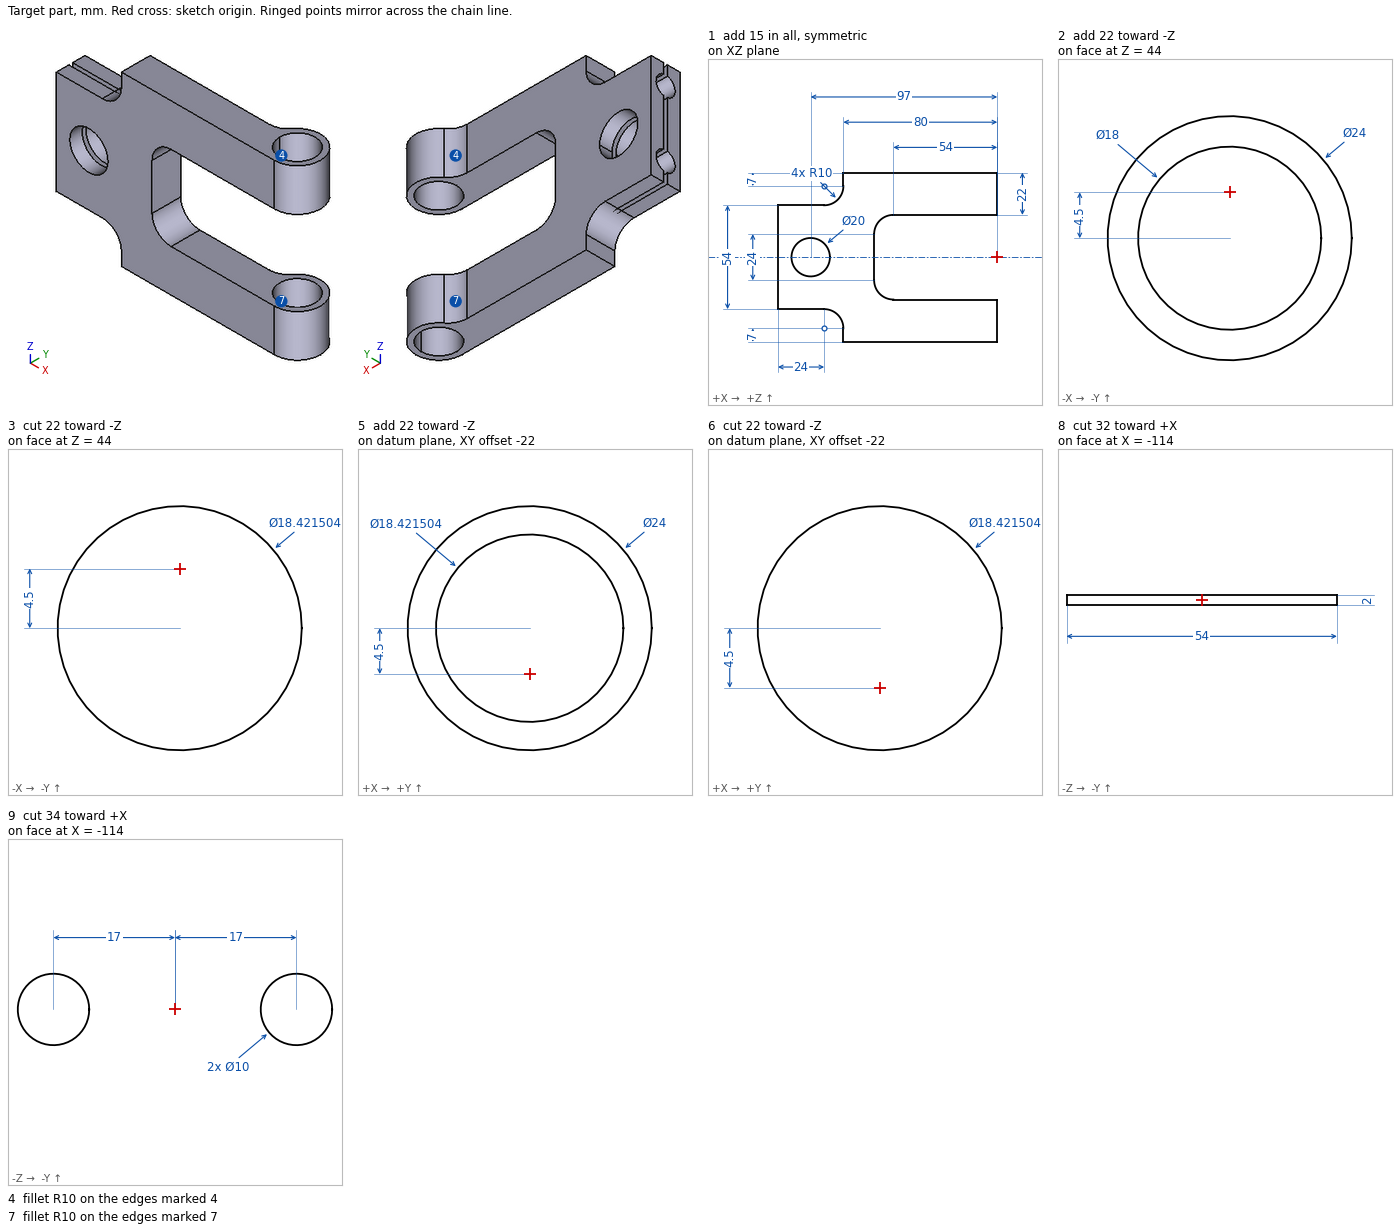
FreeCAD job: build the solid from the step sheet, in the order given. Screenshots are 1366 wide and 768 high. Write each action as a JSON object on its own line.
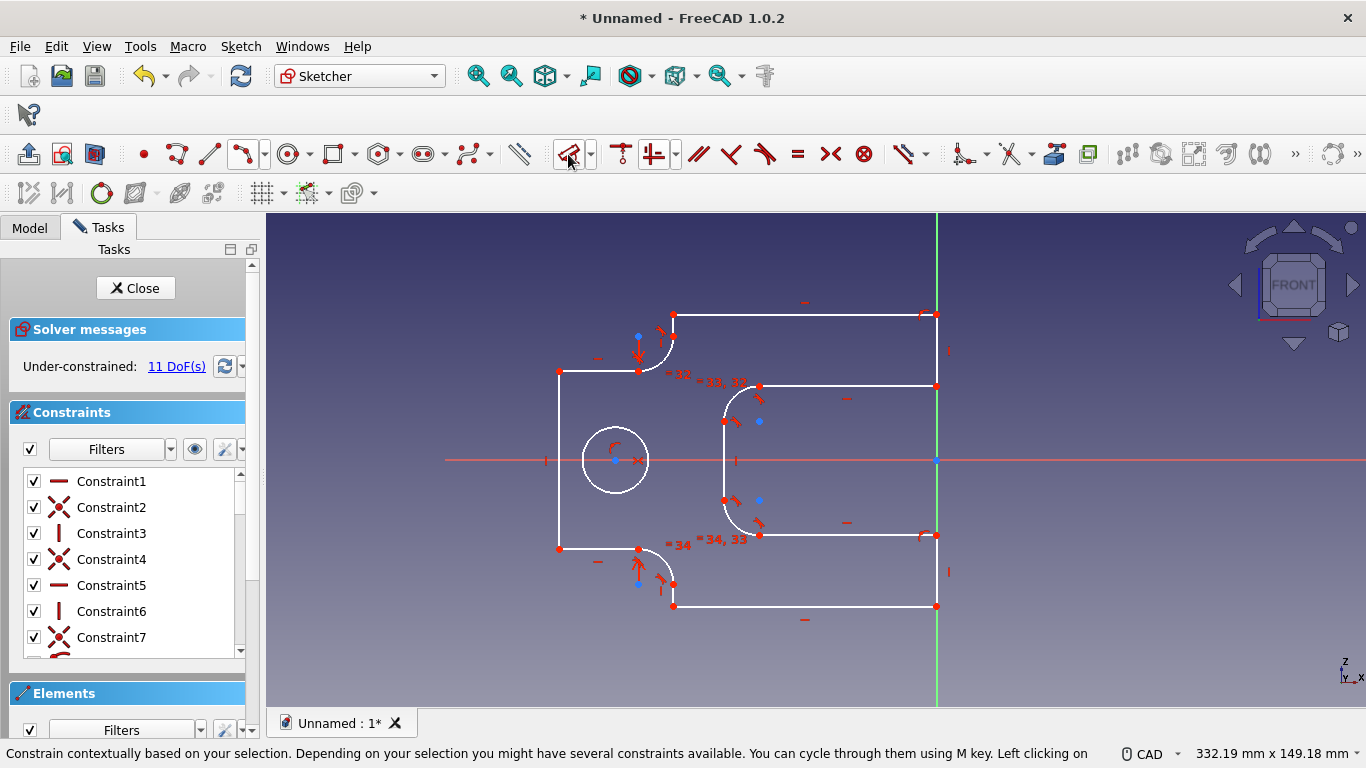
{"action": "left_click", "coordinate": [654, 367]}
{"action": "left_click", "coordinate": [668, 396]}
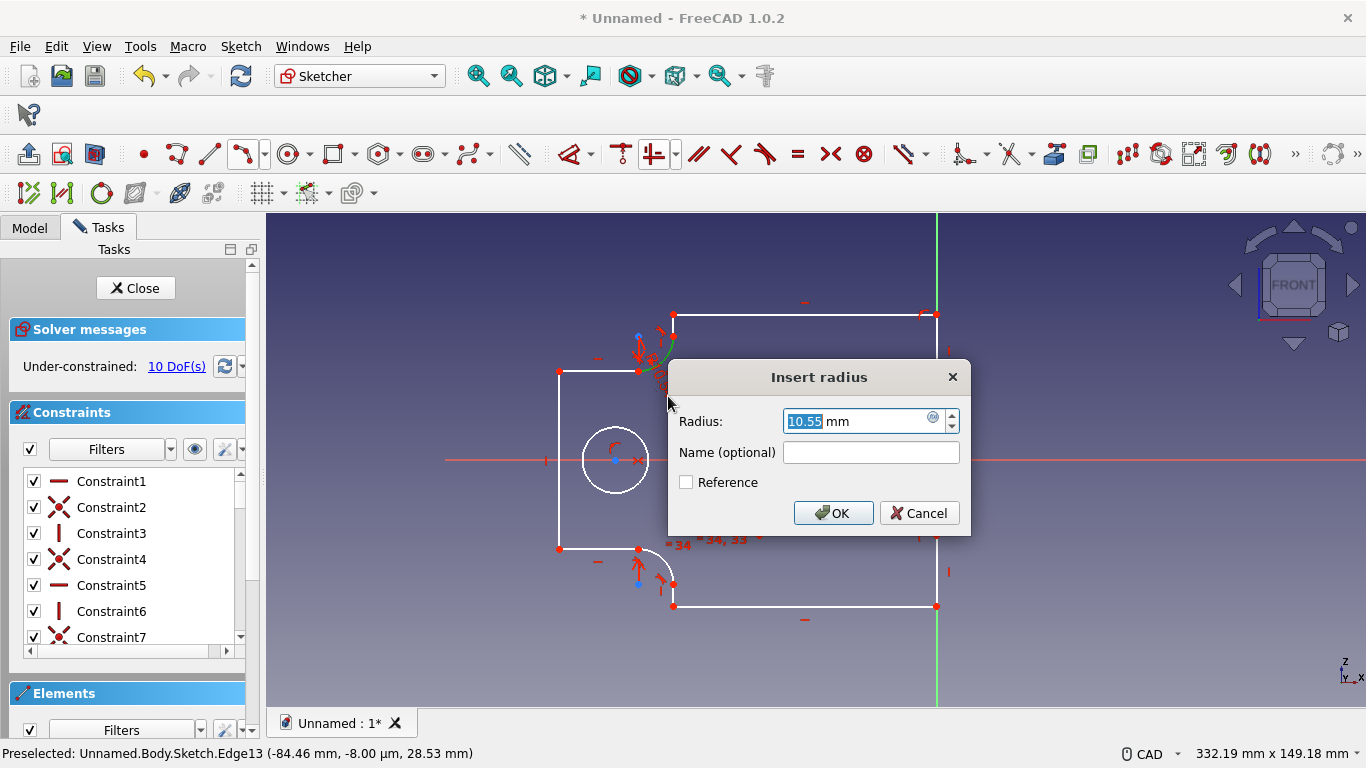
{"action": "type", "text": "10"}
{"action": "key", "text": "Return"}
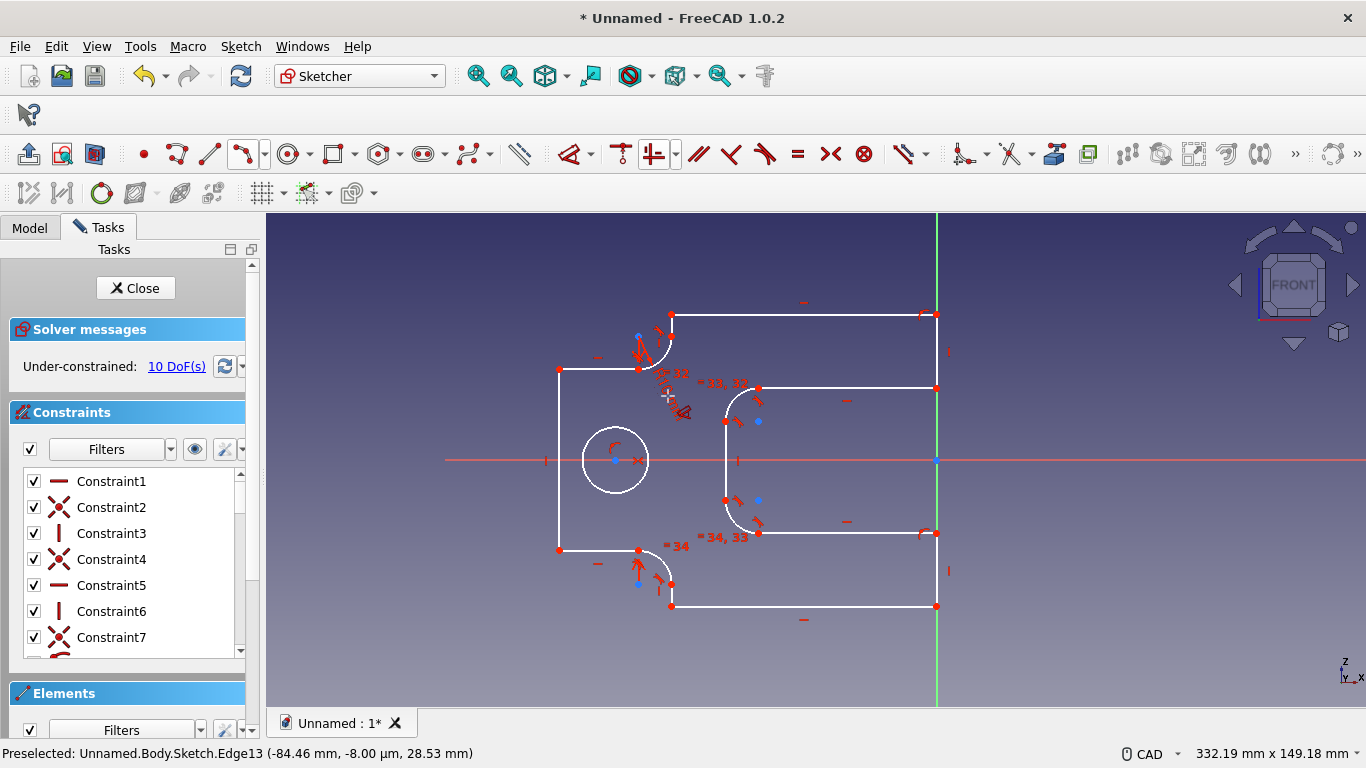
{"action": "left_click", "coordinate": [639, 437]}
{"action": "left_click", "coordinate": [678, 442]}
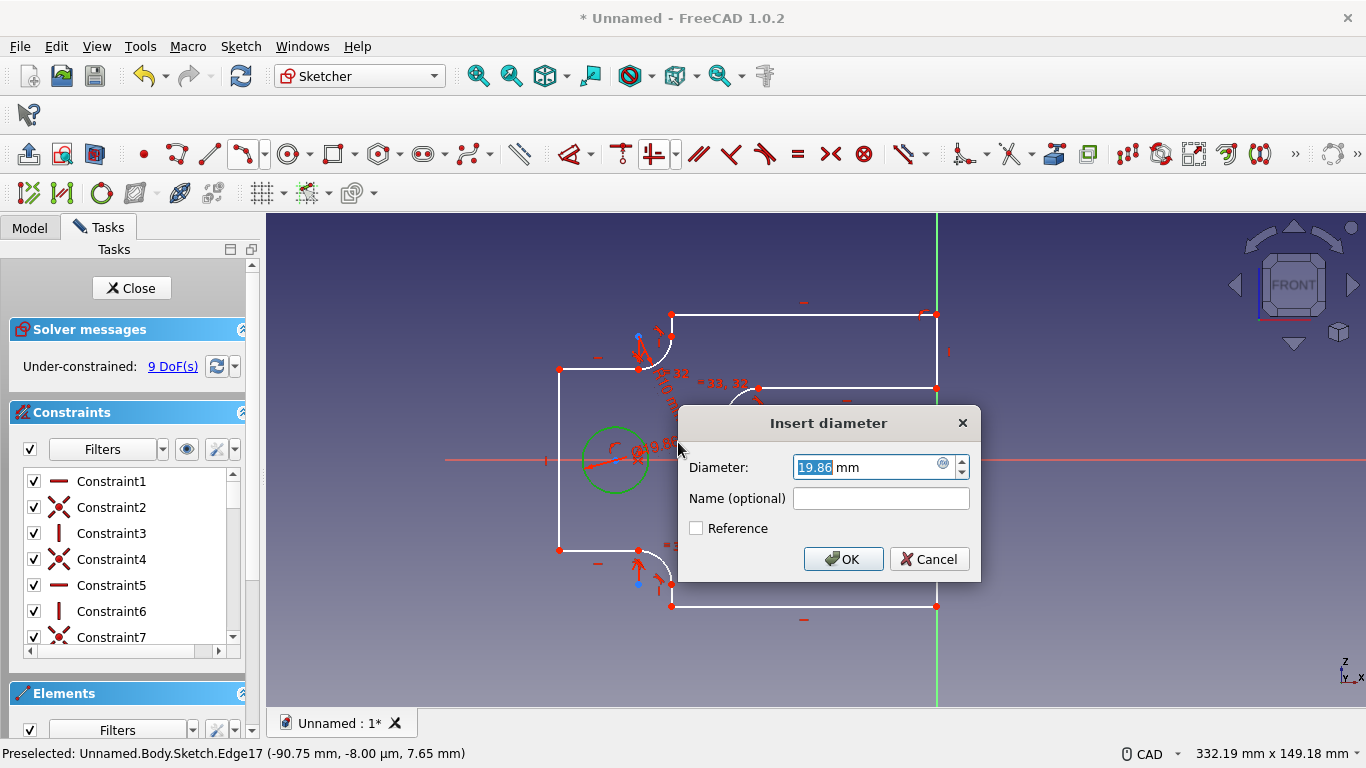
{"action": "type", "text": "20"}
{"action": "key", "text": "Return"}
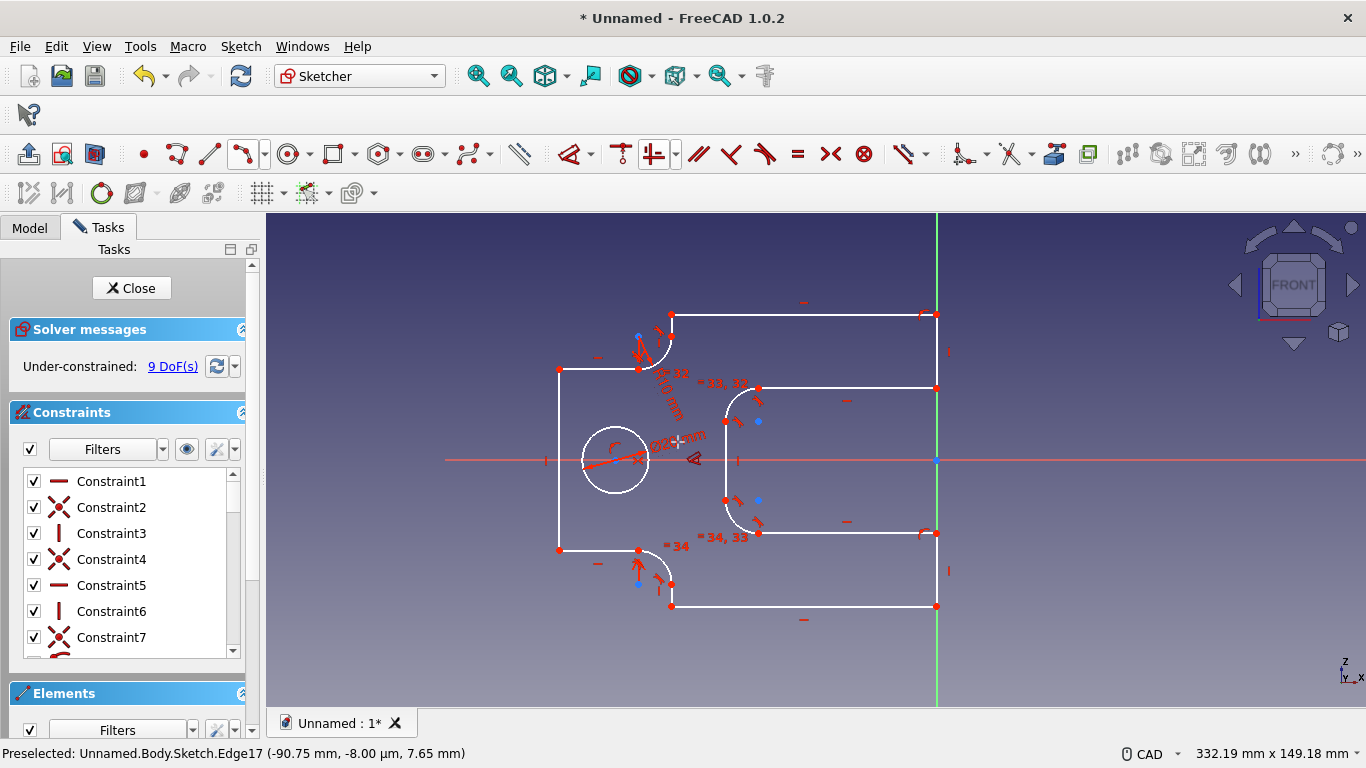
{"action": "scroll", "coordinate": [672, 326], "scroll_direction": "up", "scroll_amount": 3}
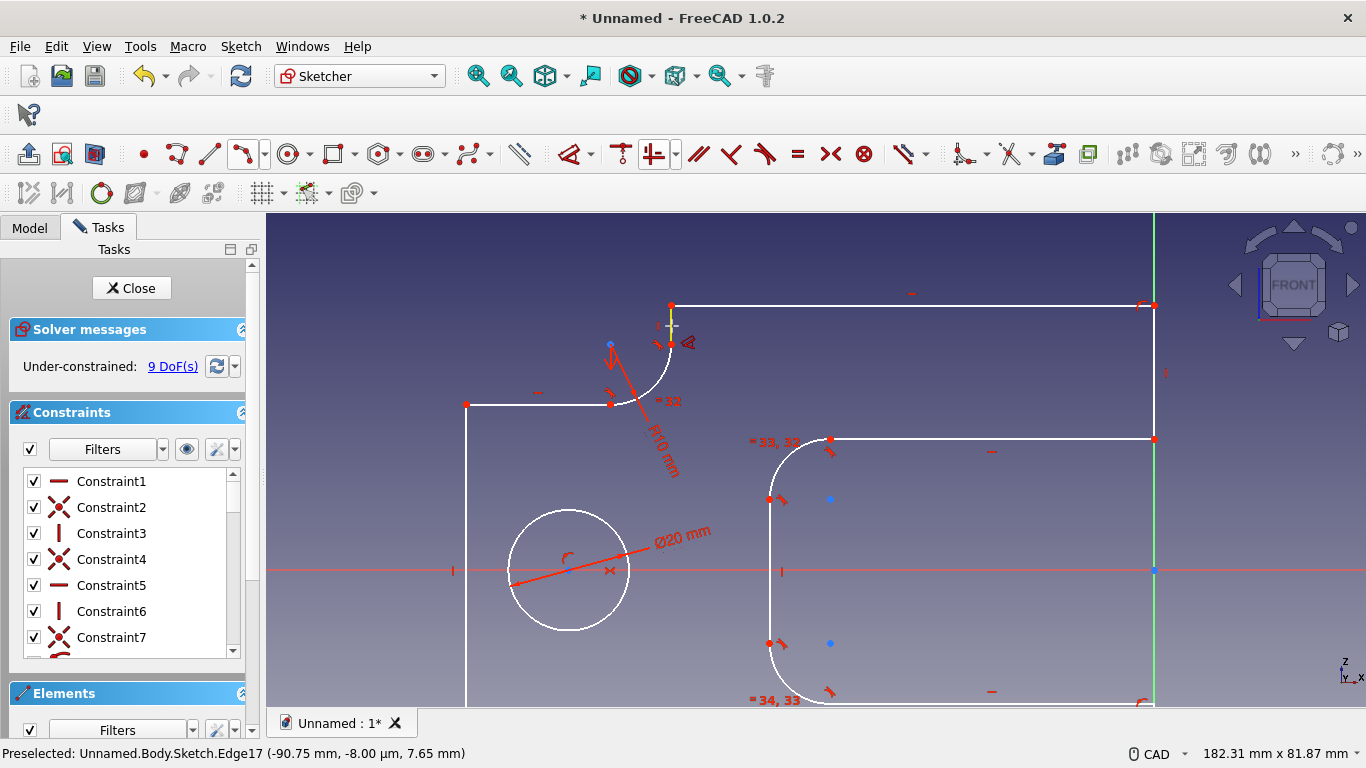
{"action": "left_click", "coordinate": [671, 325]}
{"action": "left_click", "coordinate": [637, 325]}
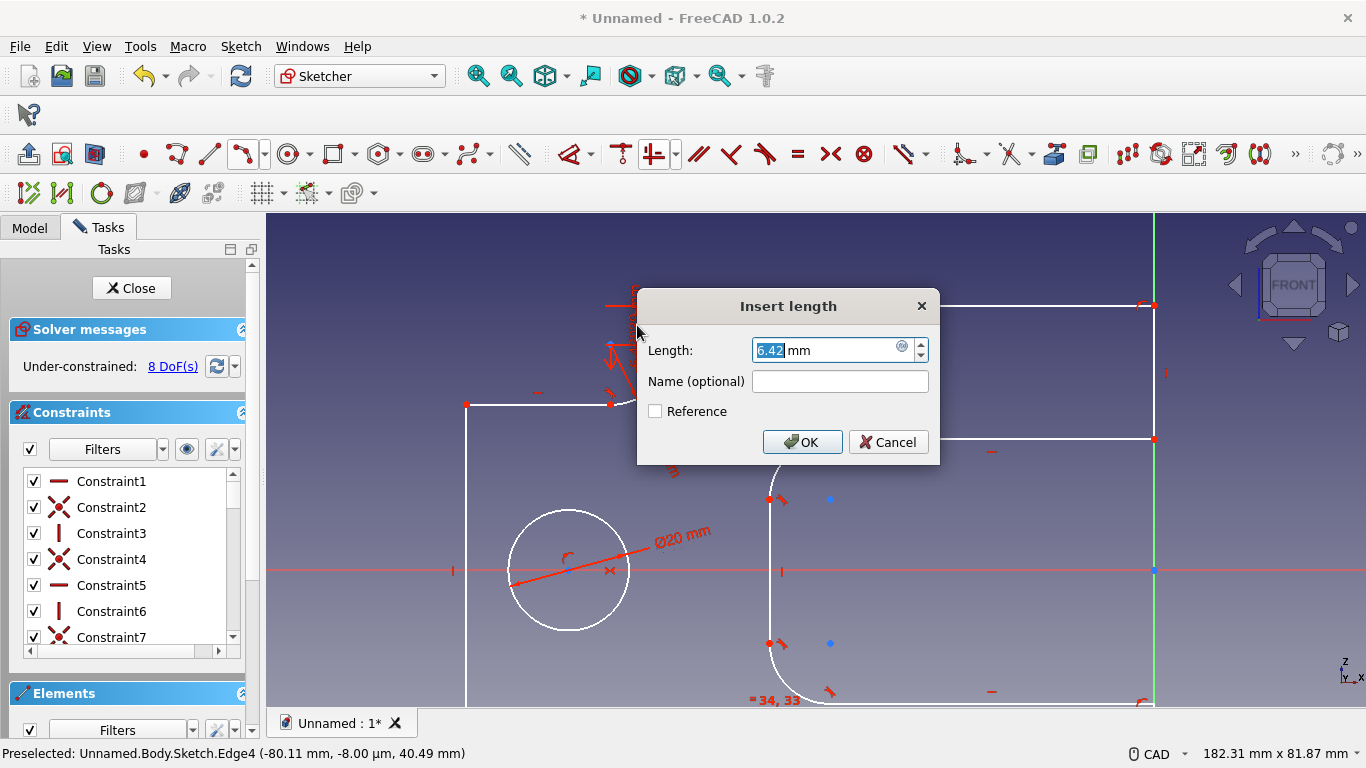
{"action": "type", "text": "7"}
{"action": "key", "text": "Return"}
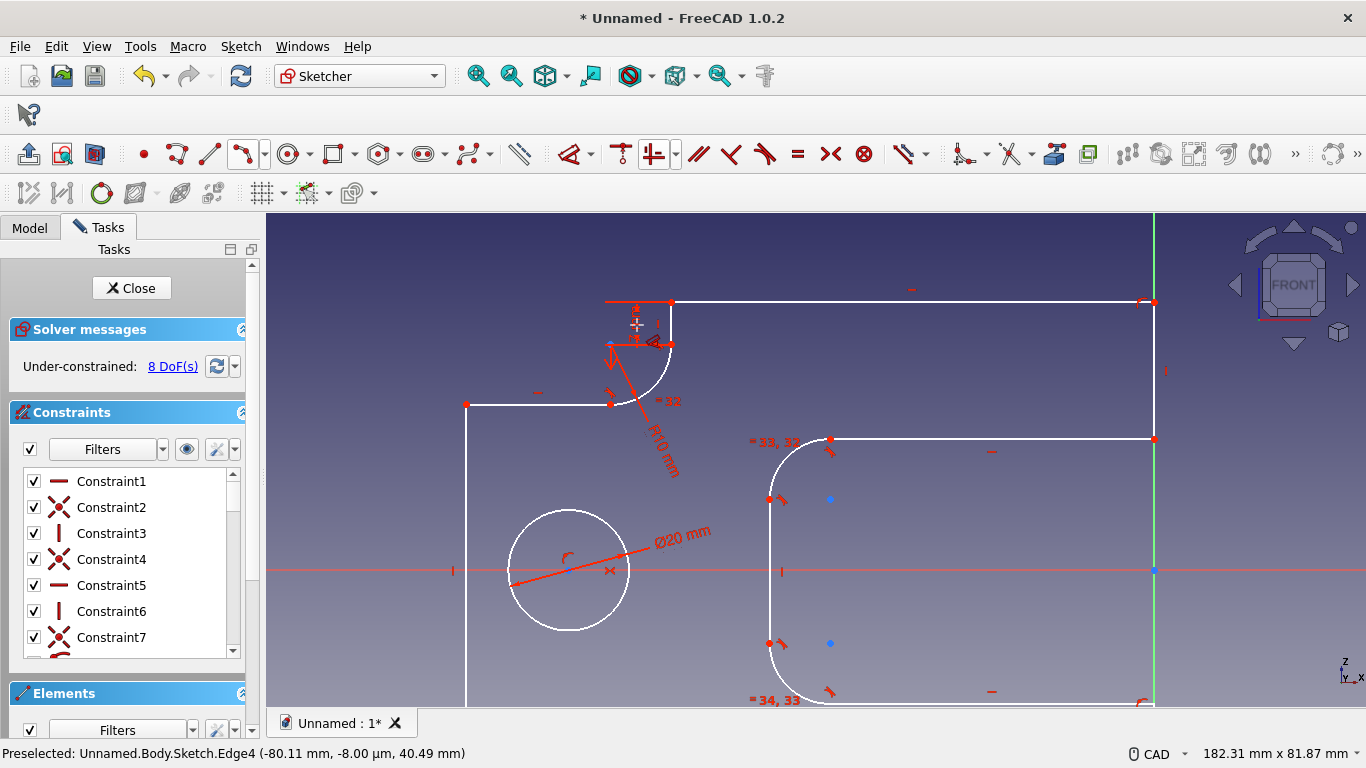
{"action": "scroll", "coordinate": [671, 326], "scroll_direction": "down", "scroll_amount": 3}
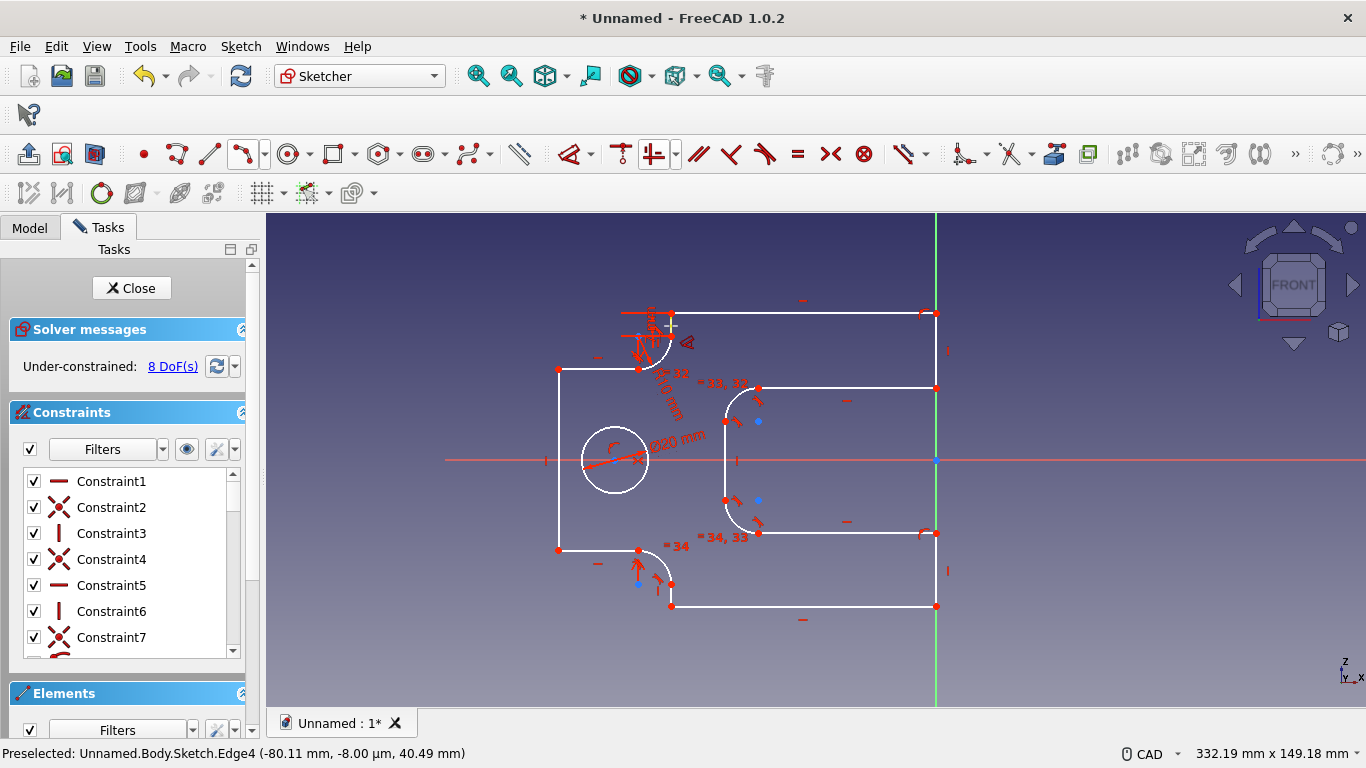
{"action": "scroll", "coordinate": [671, 600], "scroll_direction": "up", "scroll_amount": 4}